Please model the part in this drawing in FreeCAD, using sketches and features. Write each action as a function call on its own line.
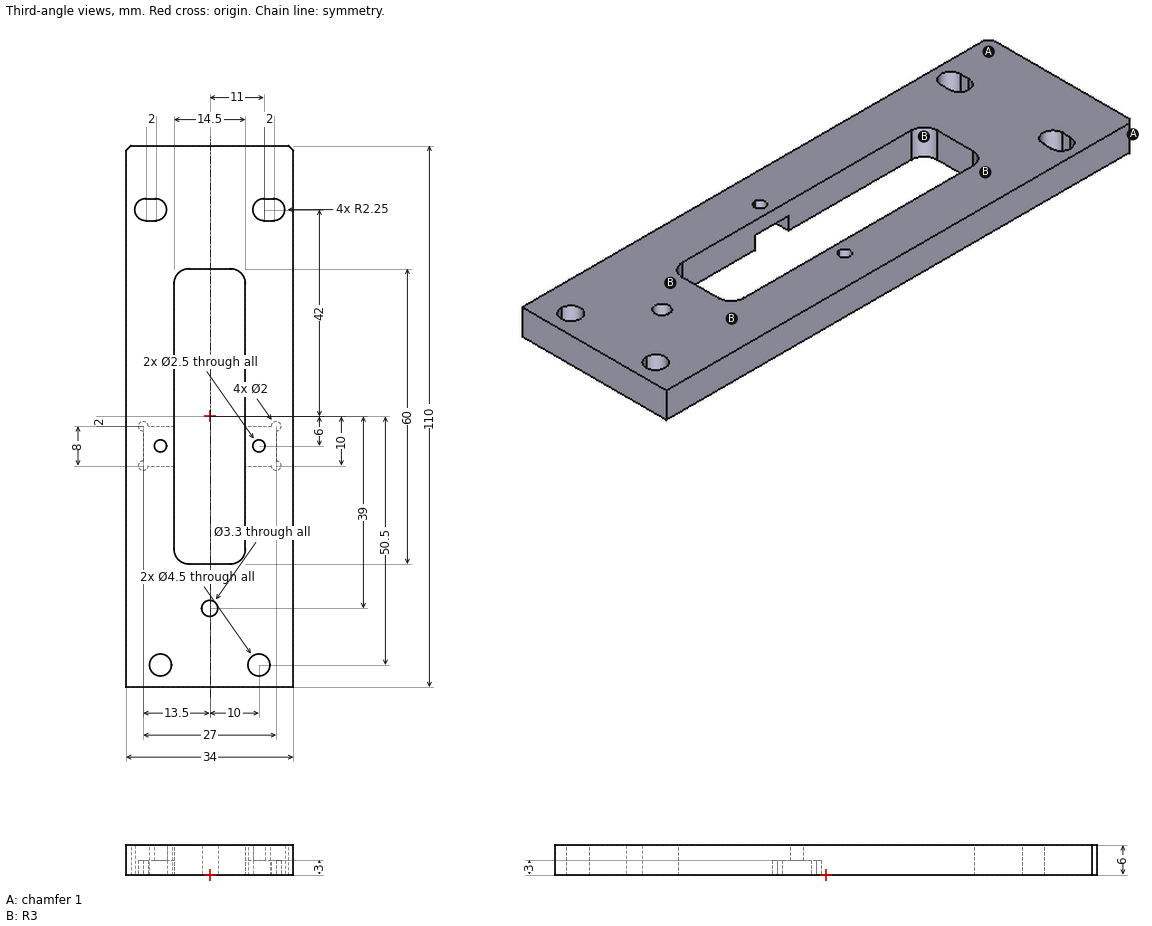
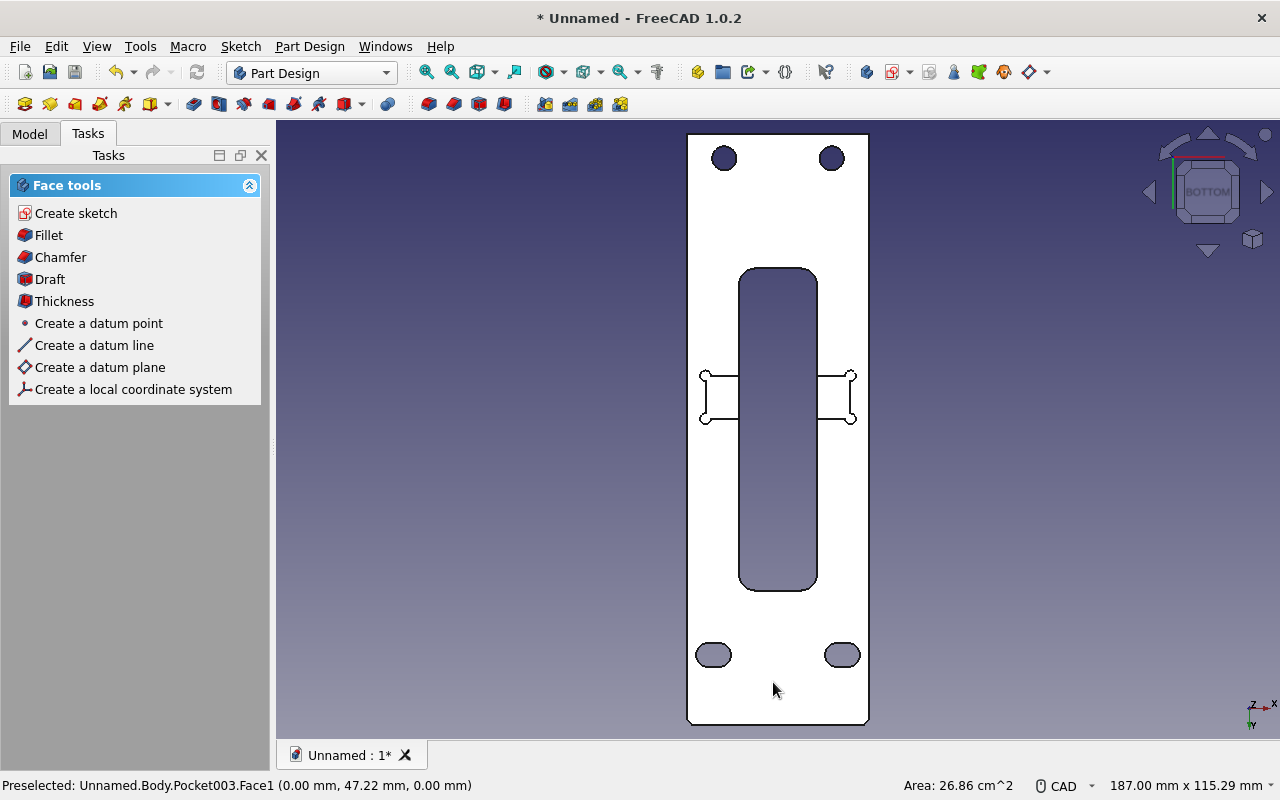
click(892, 72)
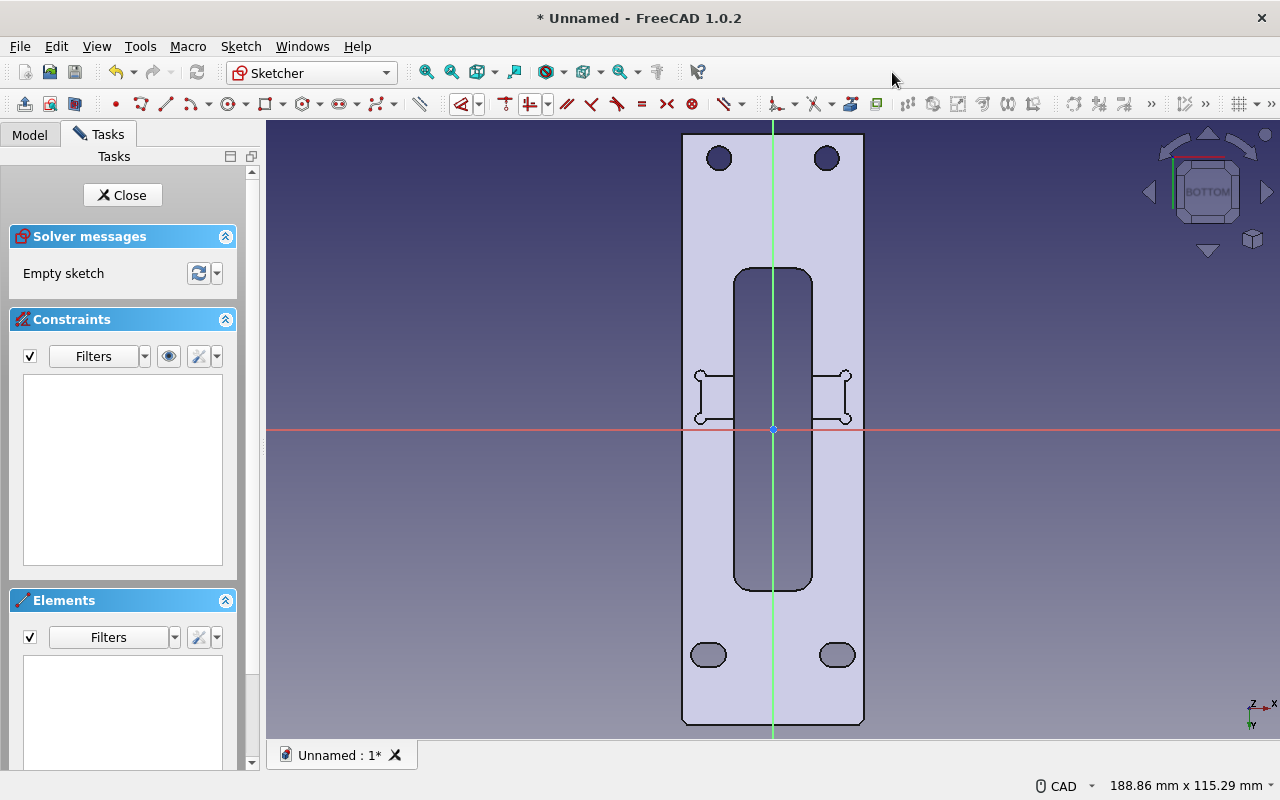
scroll(790, 405, up, 8)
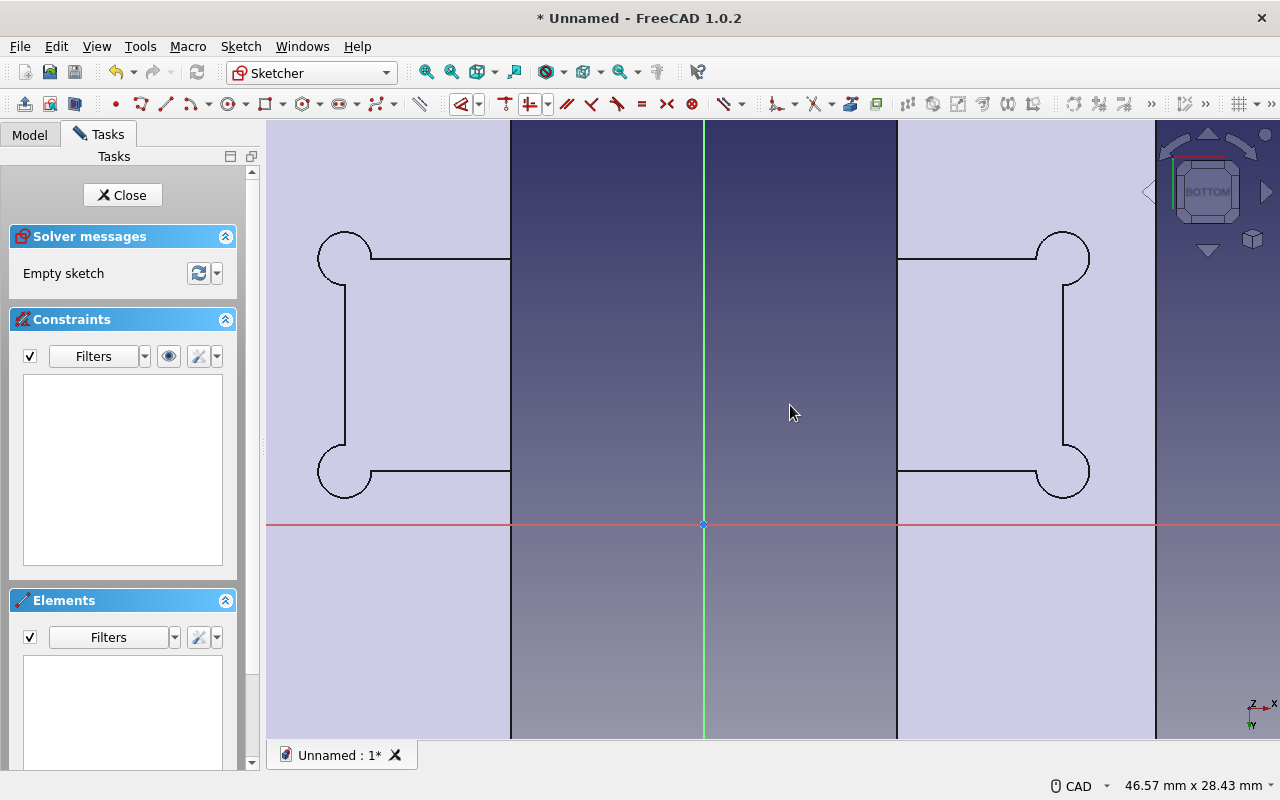
click(228, 104)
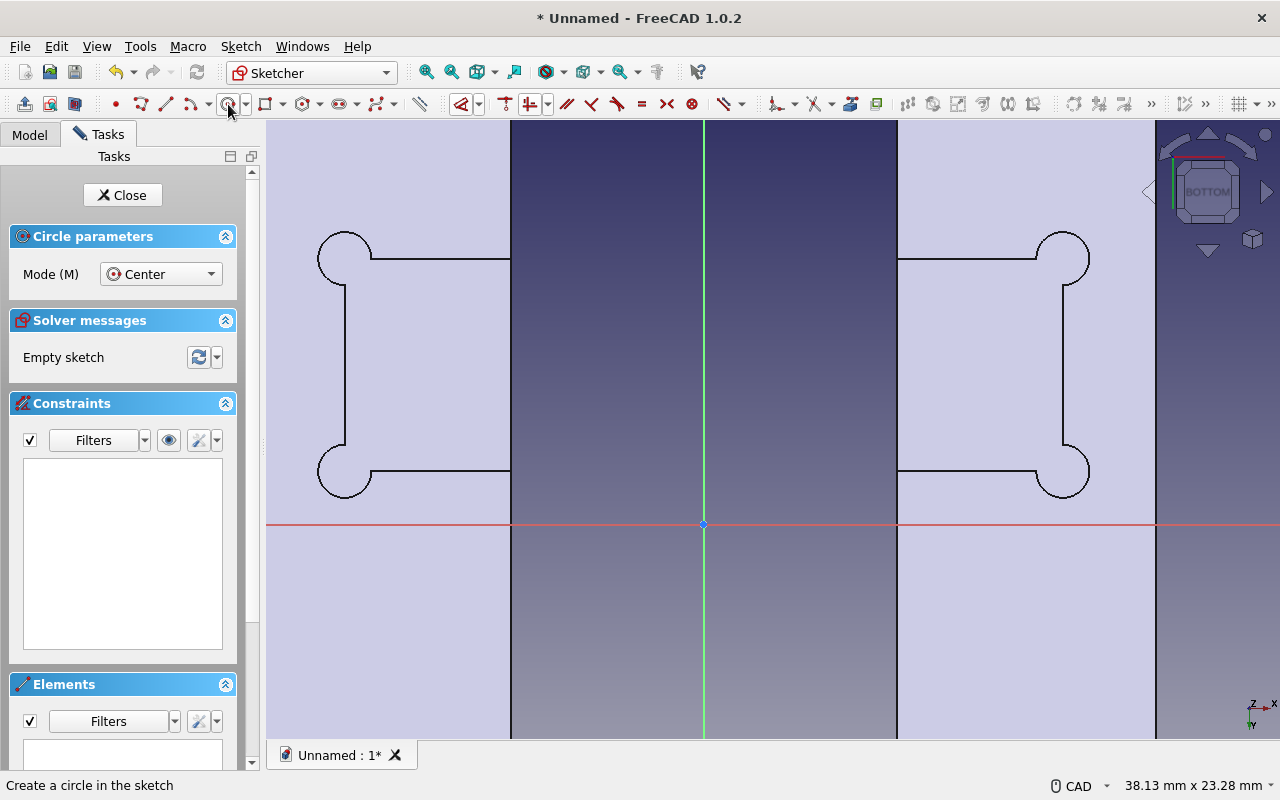
click(970, 365)
click(993, 341)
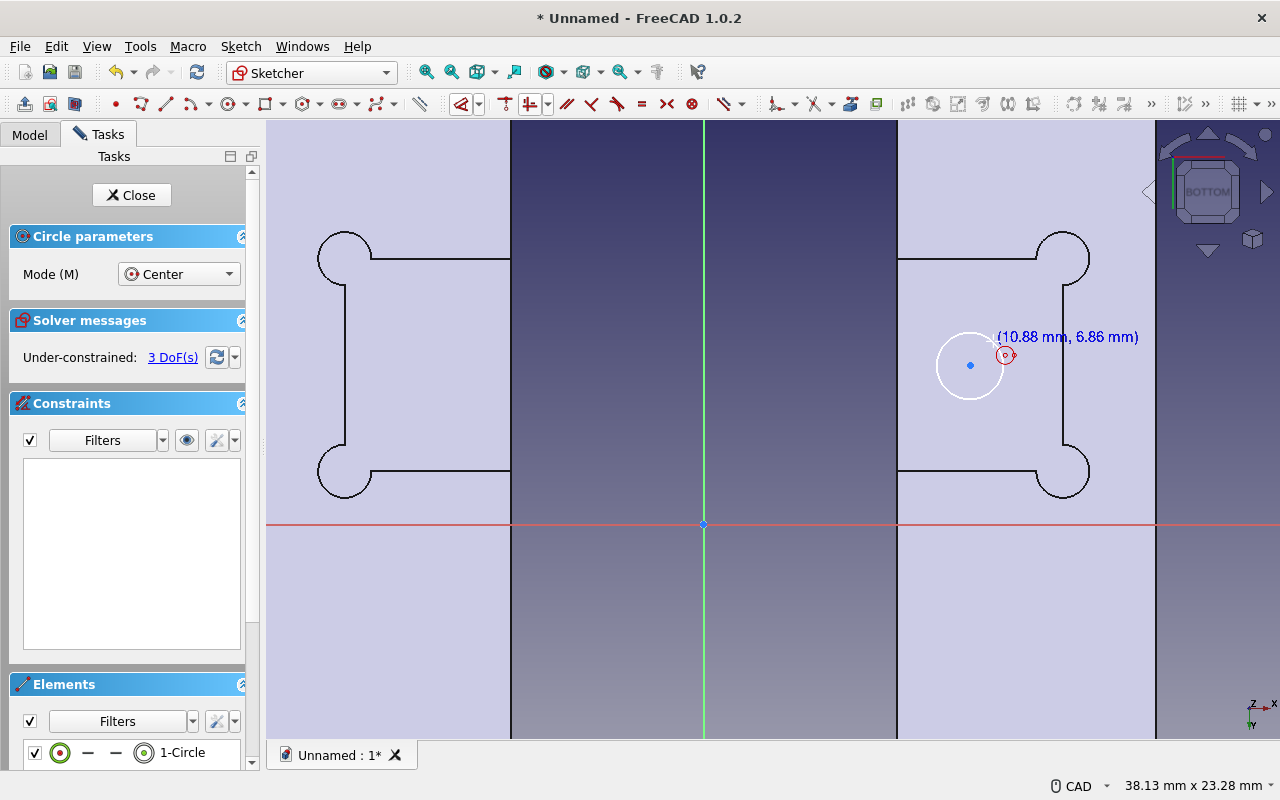
click(438, 365)
click(461, 341)
key(Escape)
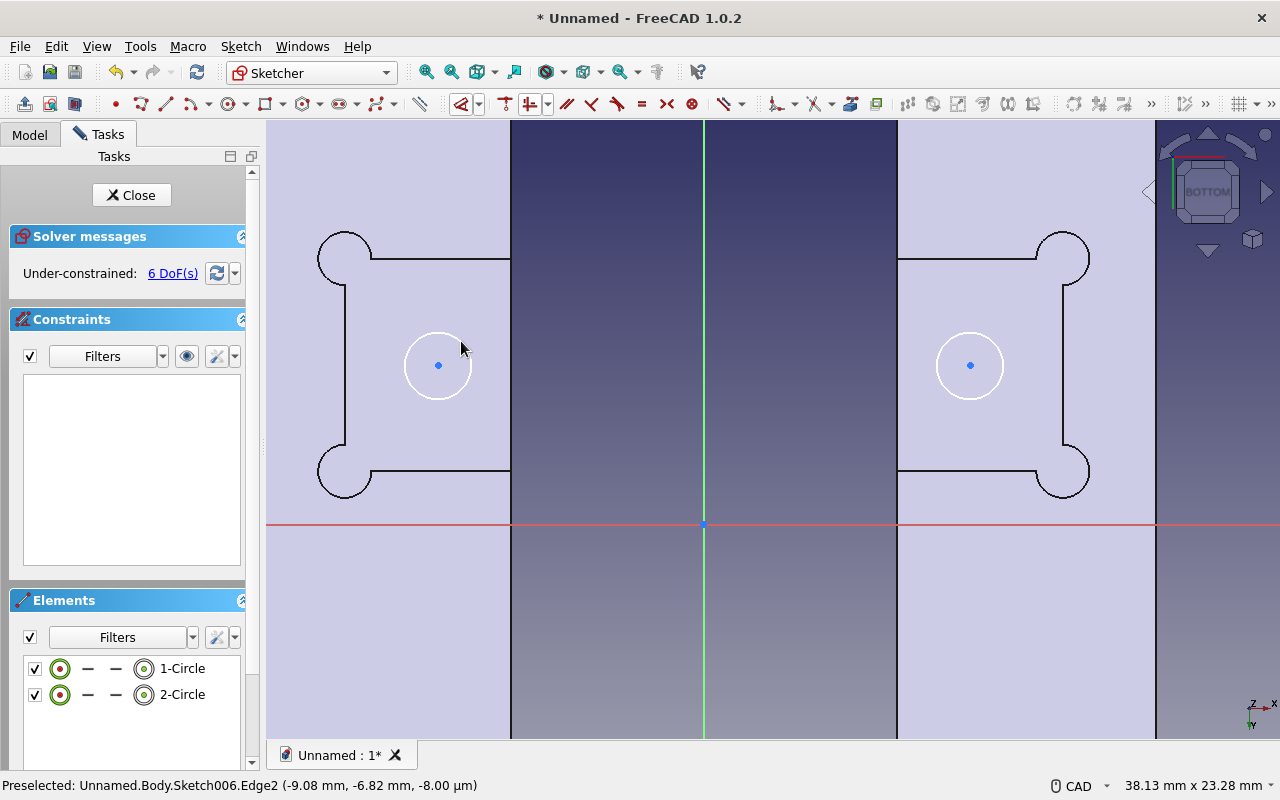
click(993, 342)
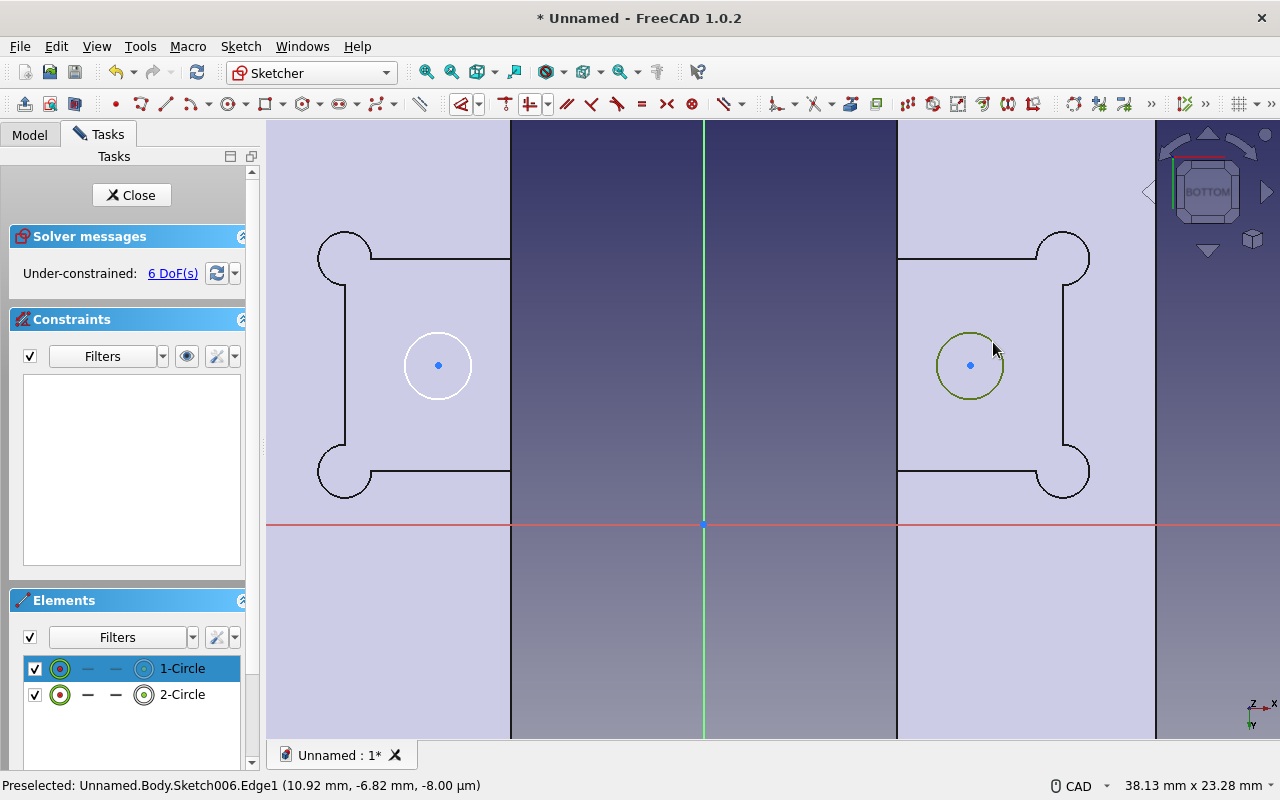
click(461, 342)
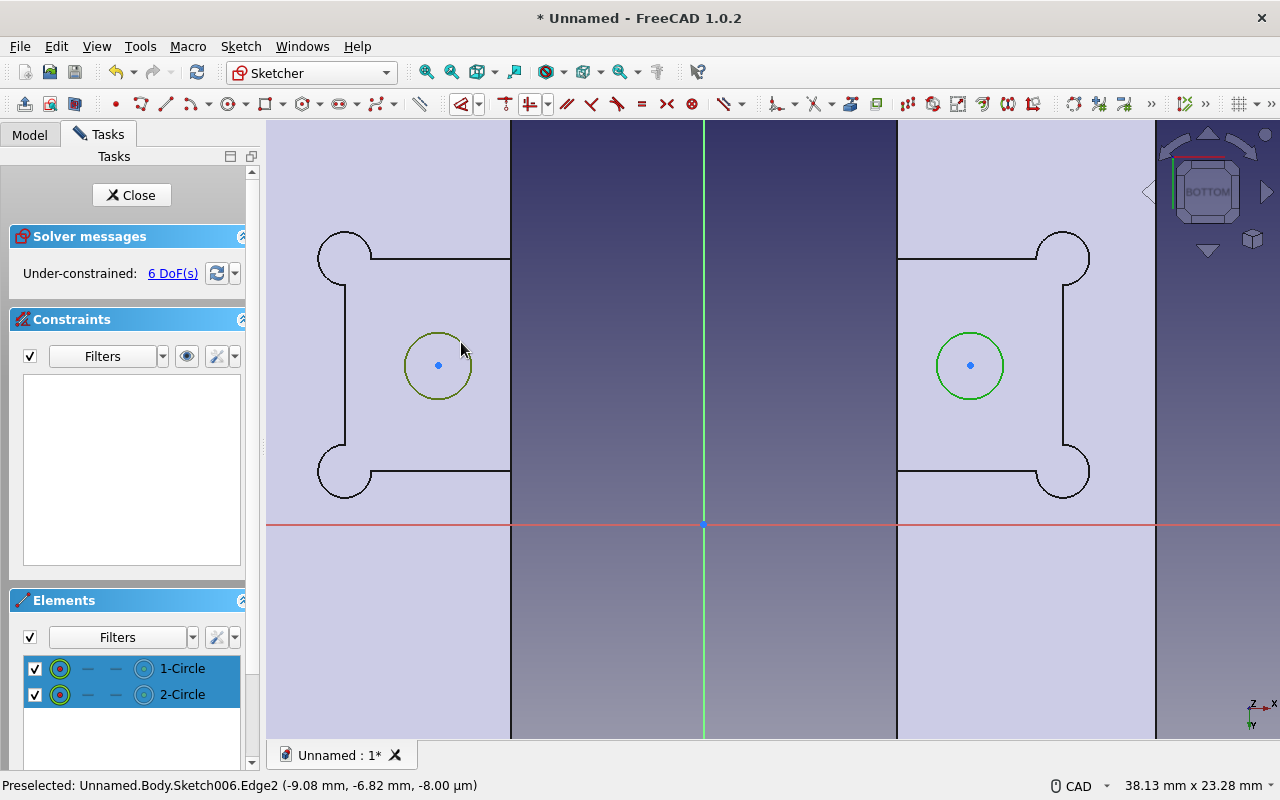
key(e)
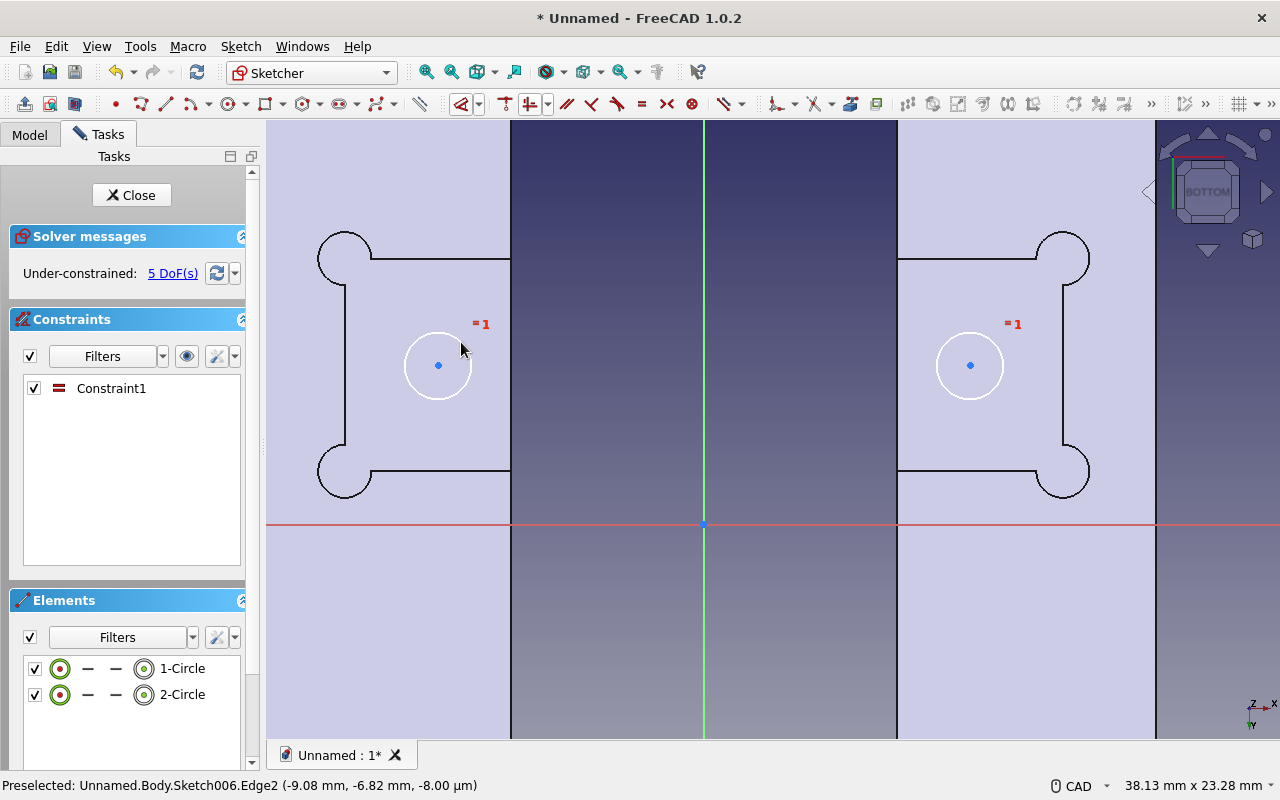
click(970, 366)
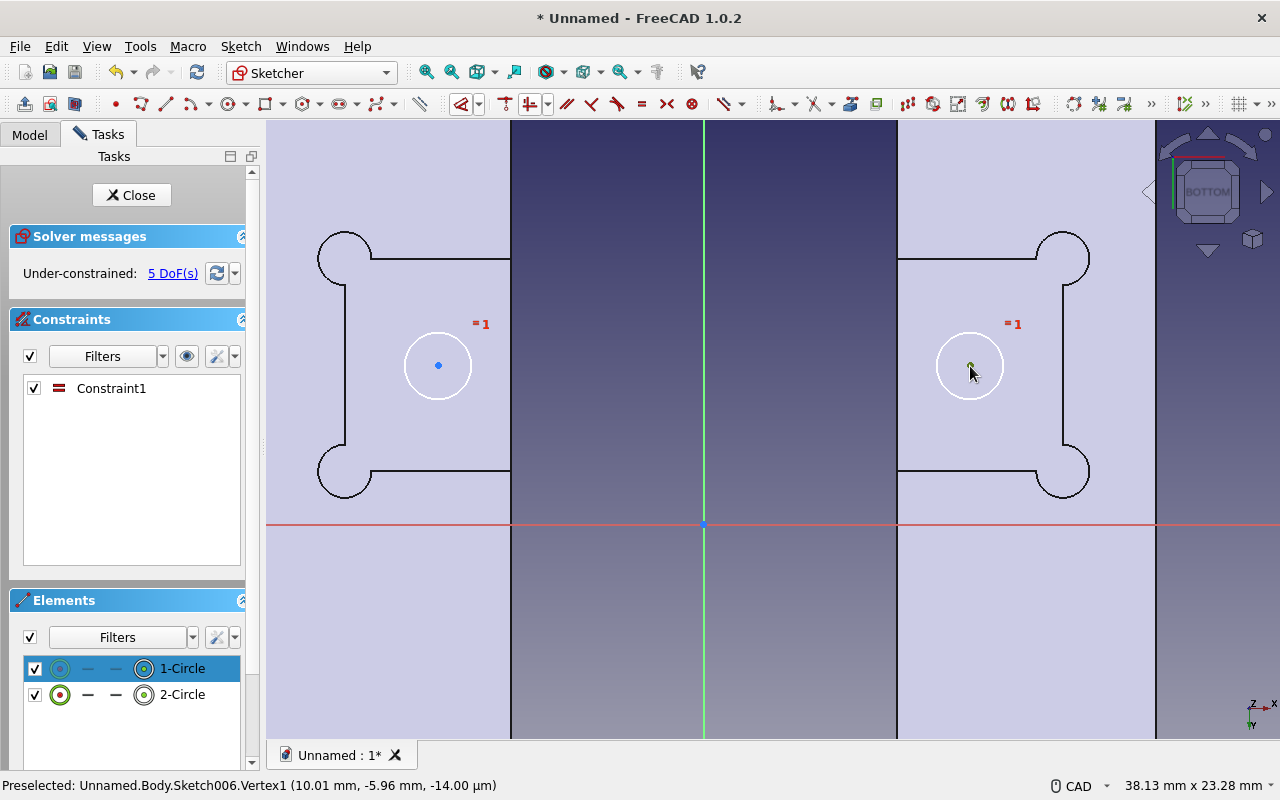
click(438, 366)